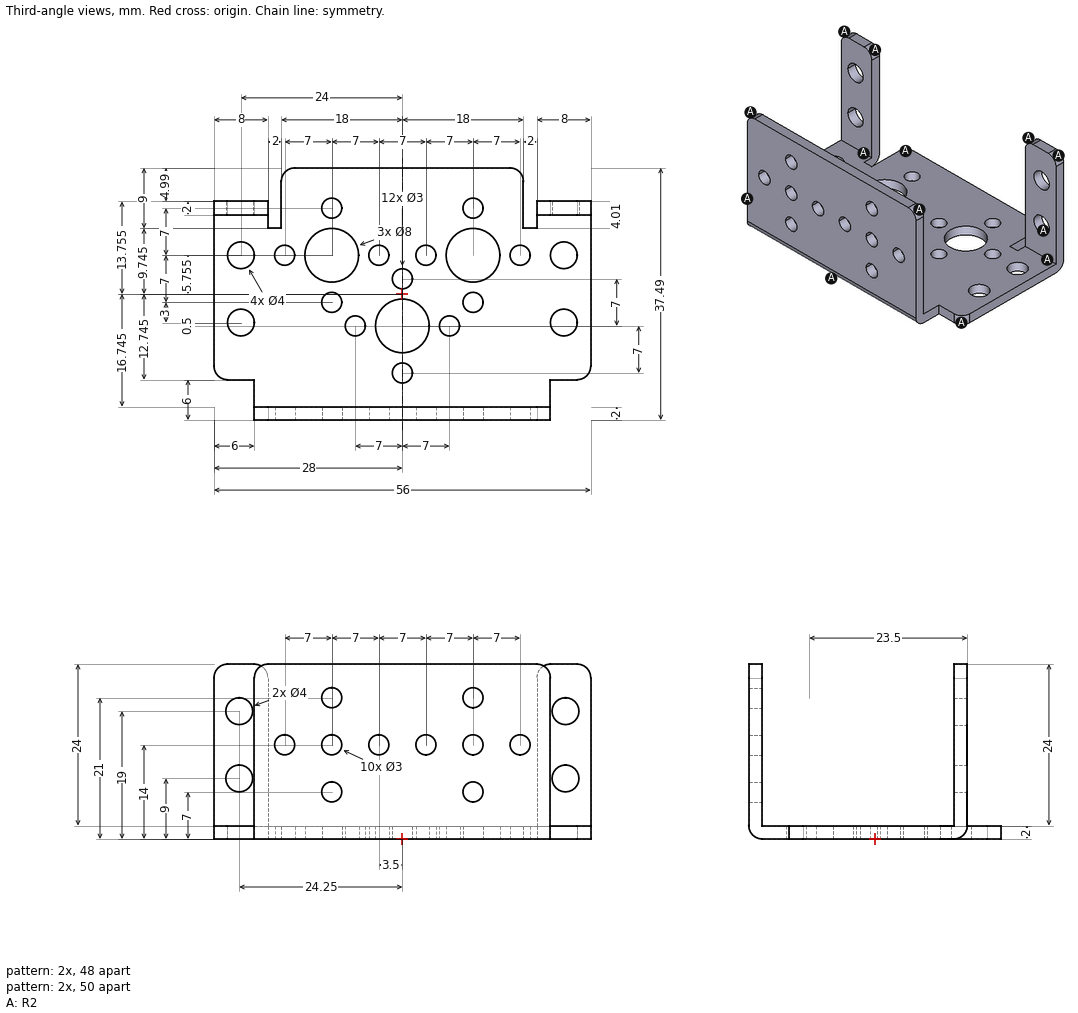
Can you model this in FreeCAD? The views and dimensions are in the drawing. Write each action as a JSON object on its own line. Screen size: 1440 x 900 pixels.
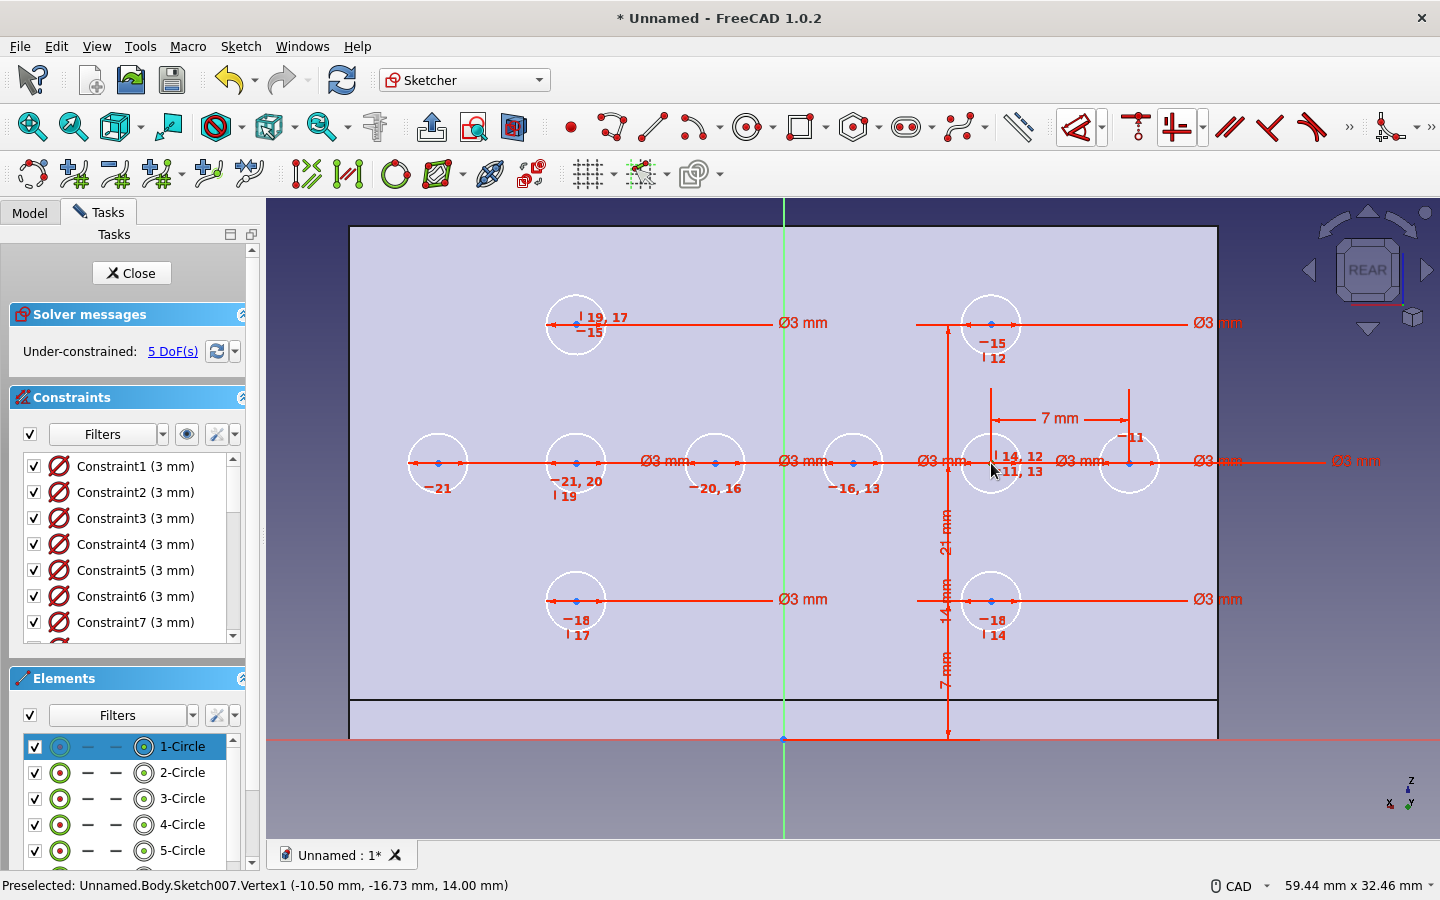
{"action": "left_click", "coordinate": [853, 463]}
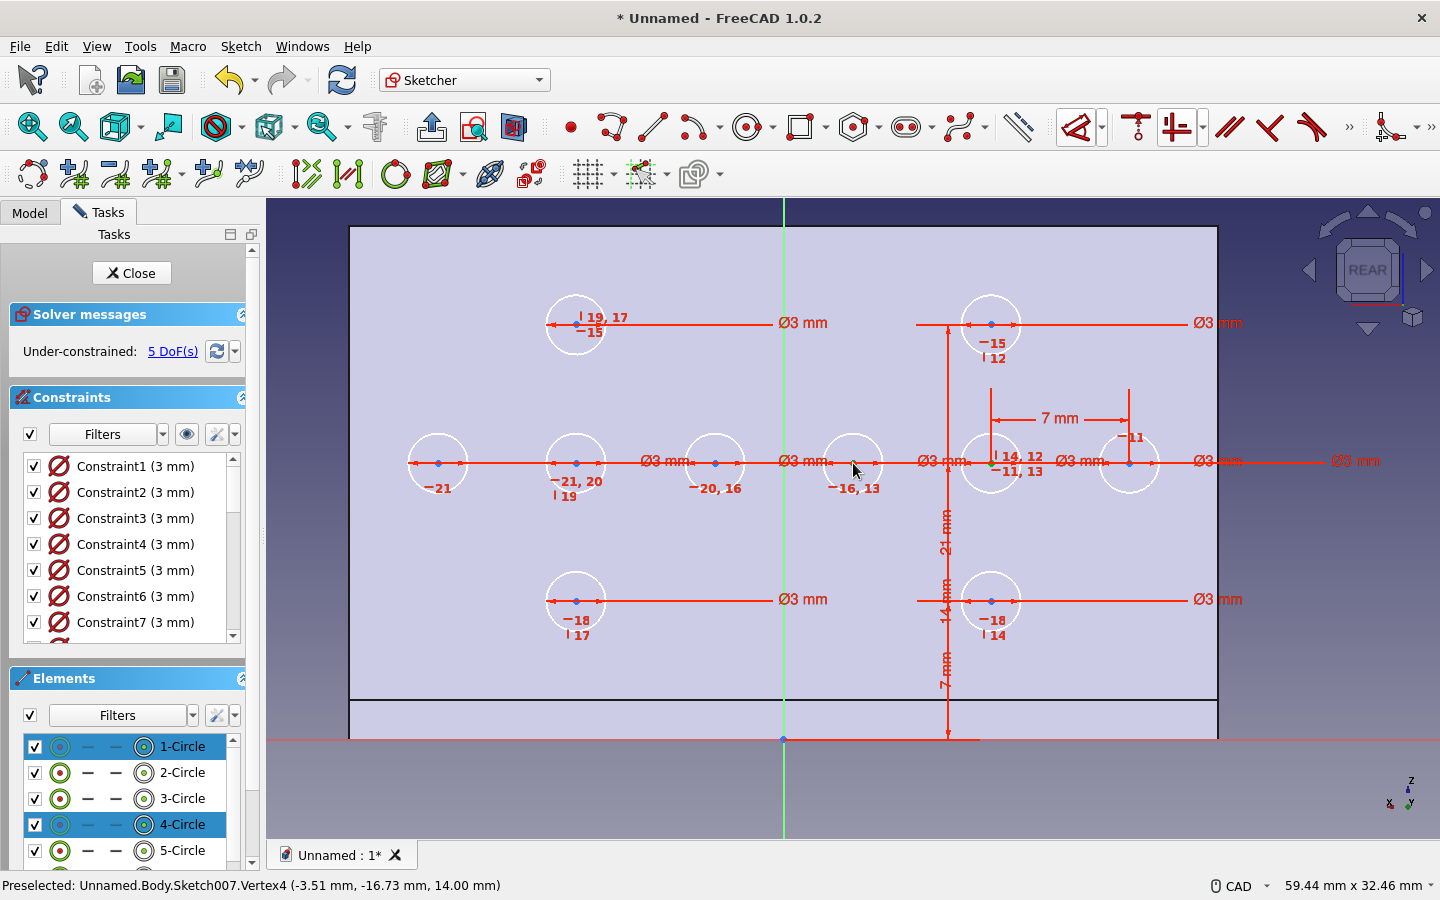
{"action": "key", "text": "l"}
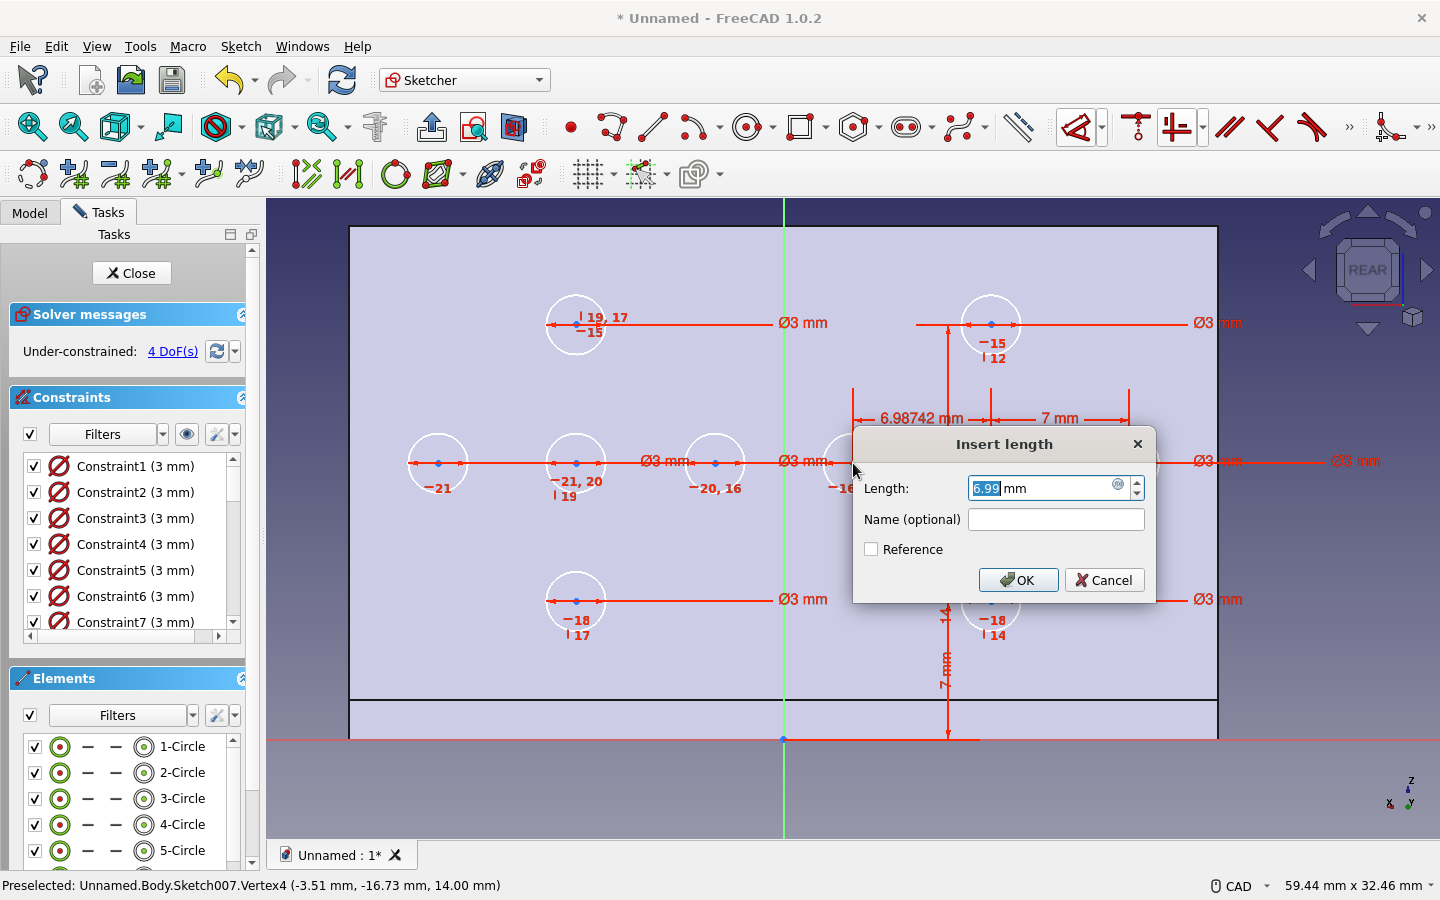
{"action": "type", "text": "7"}
{"action": "key", "text": "Return"}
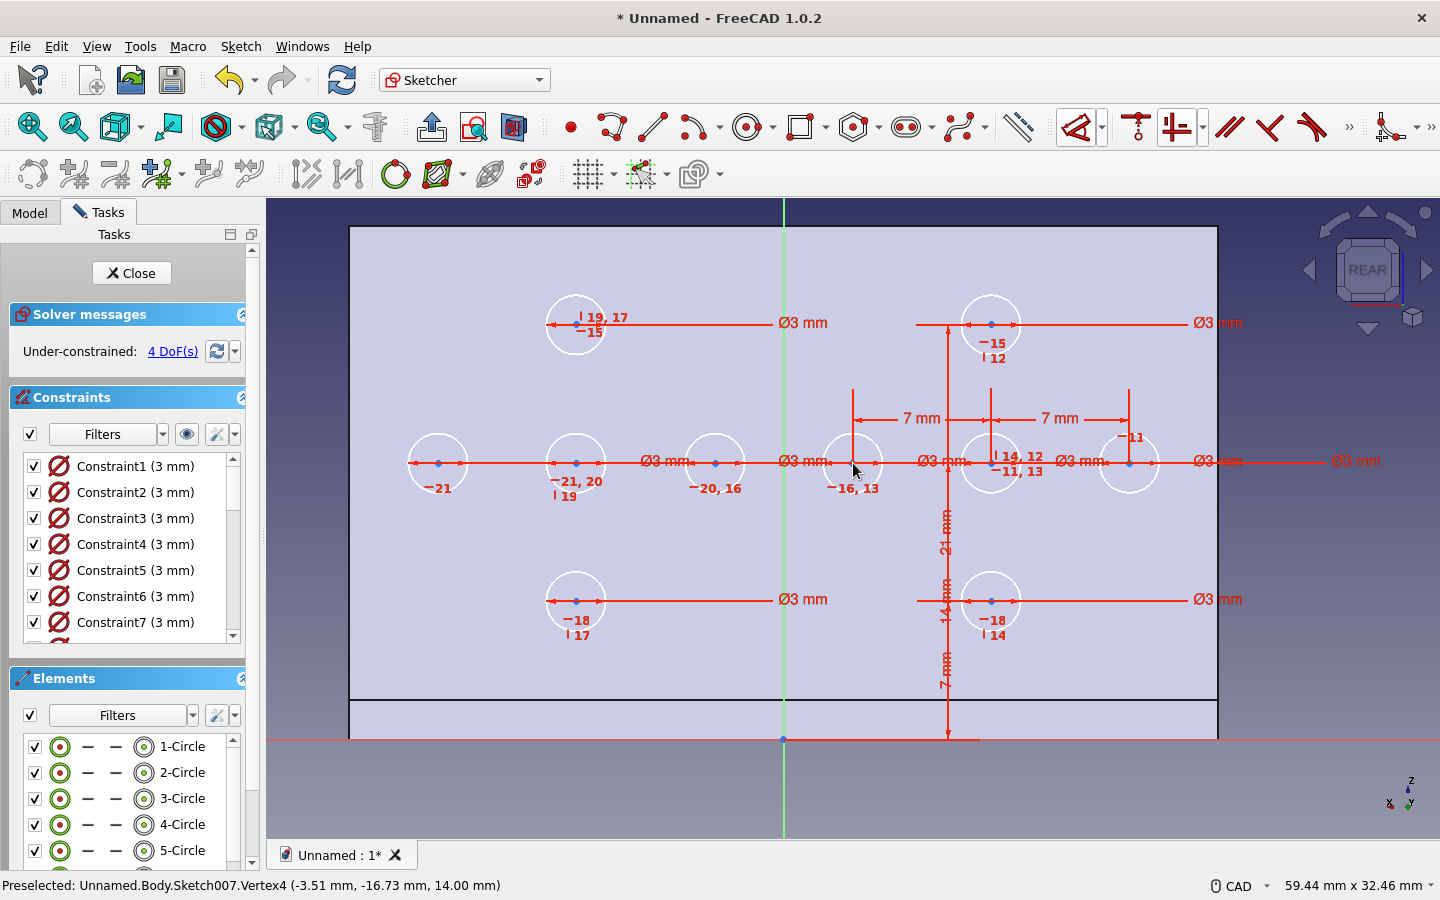
{"action": "left_click", "coordinate": [853, 463]}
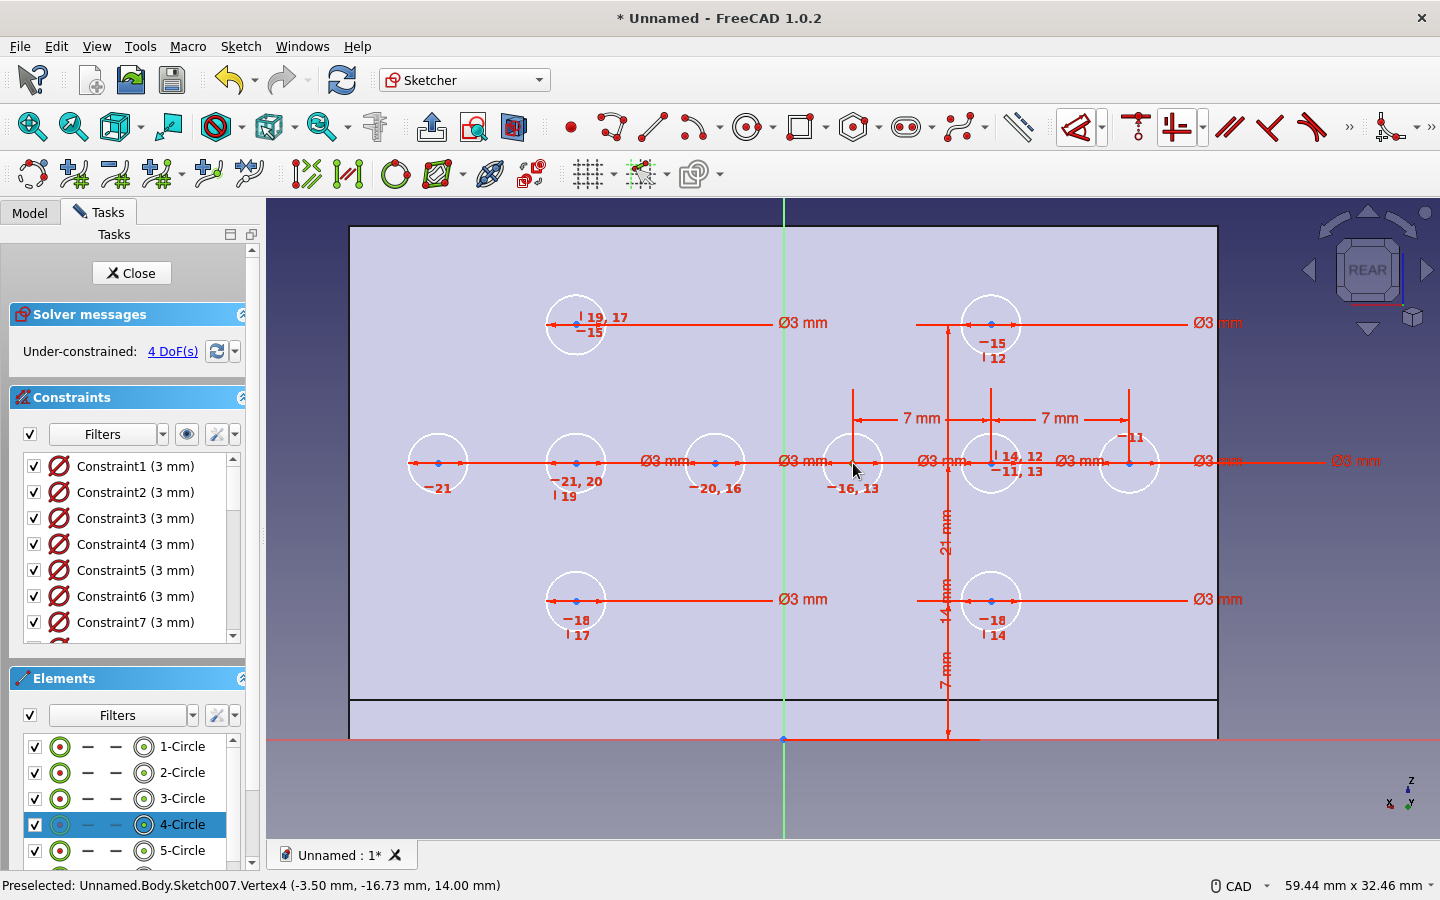
{"action": "left_click", "coordinate": [715, 463]}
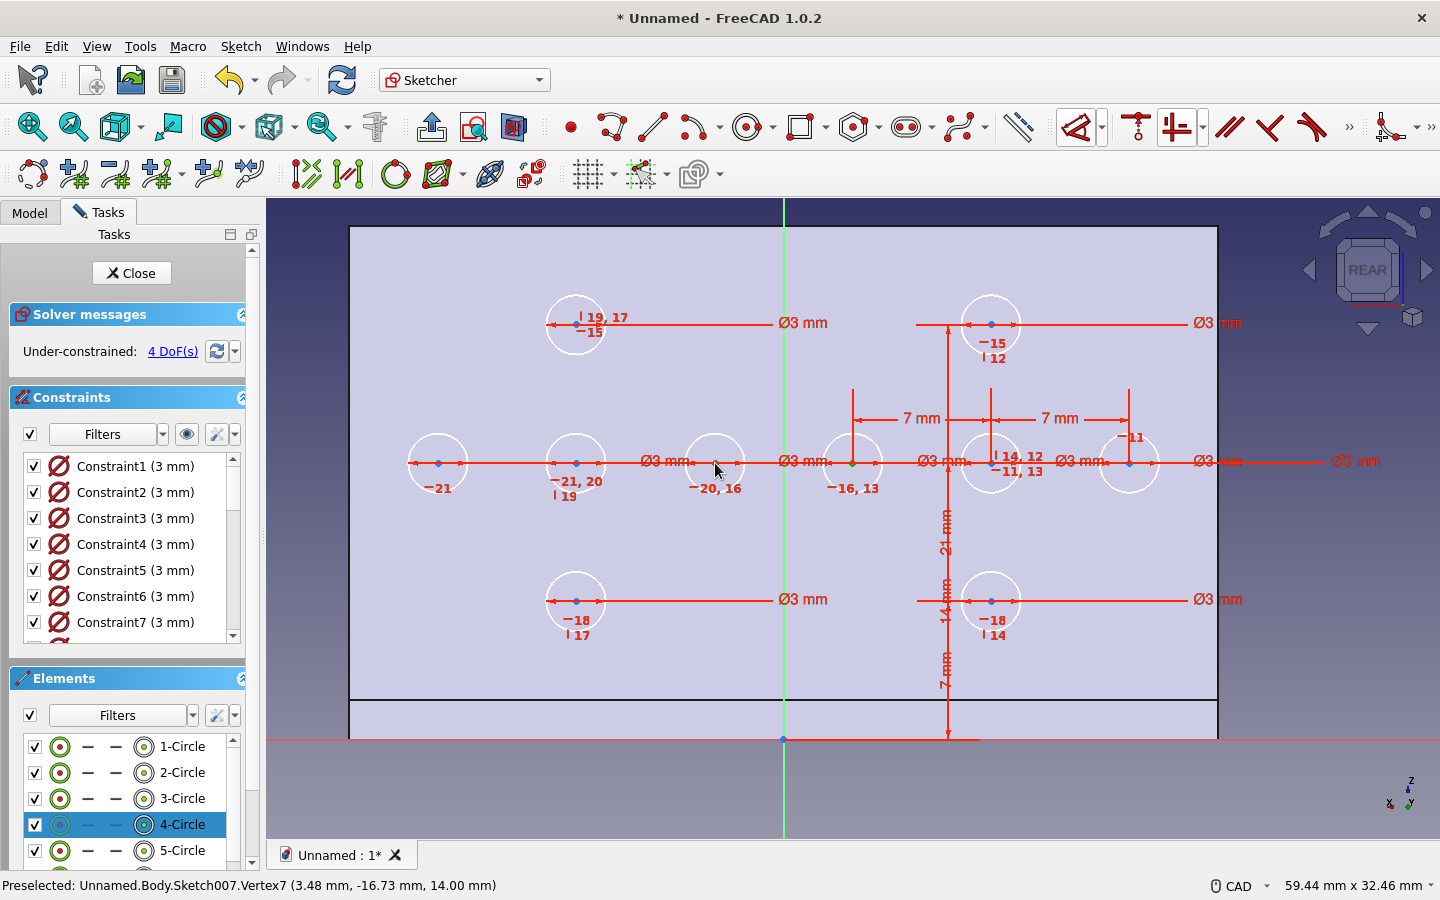
{"action": "key", "text": "l"}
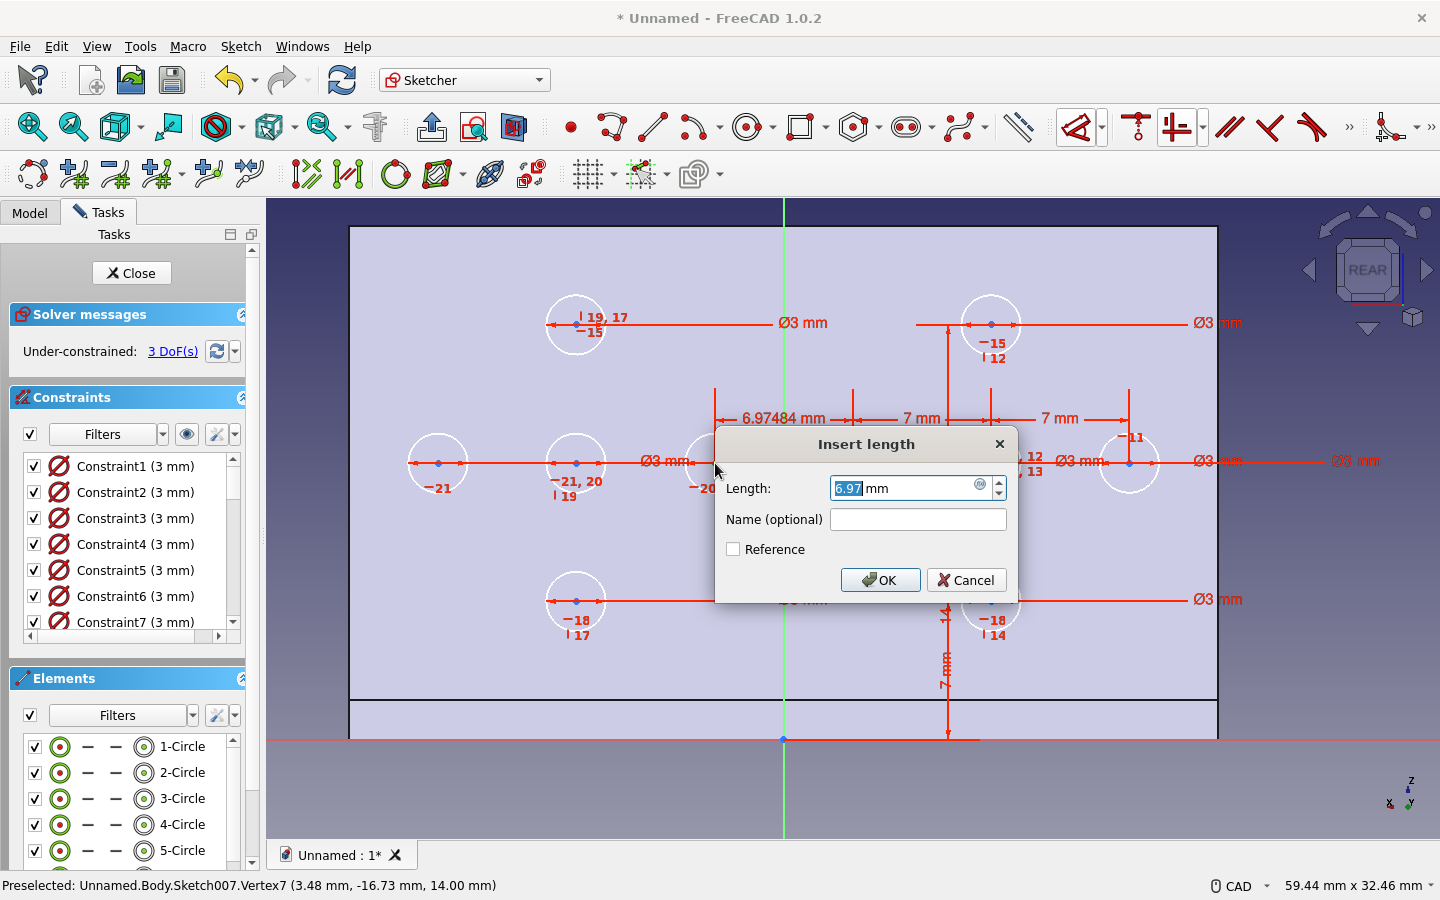
{"action": "type", "text": "7"}
{"action": "key", "text": "Return"}